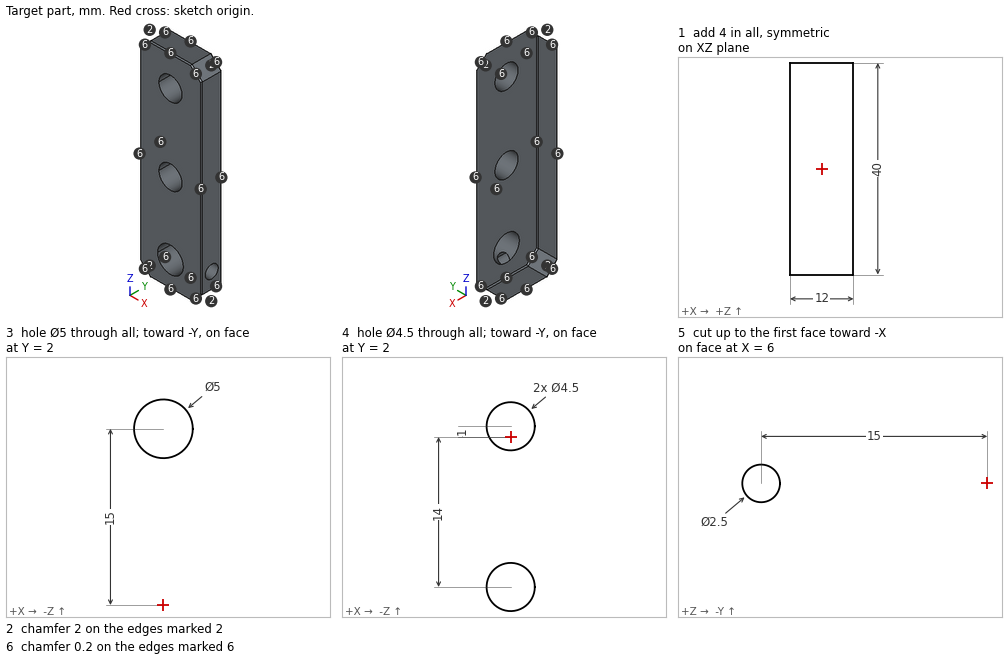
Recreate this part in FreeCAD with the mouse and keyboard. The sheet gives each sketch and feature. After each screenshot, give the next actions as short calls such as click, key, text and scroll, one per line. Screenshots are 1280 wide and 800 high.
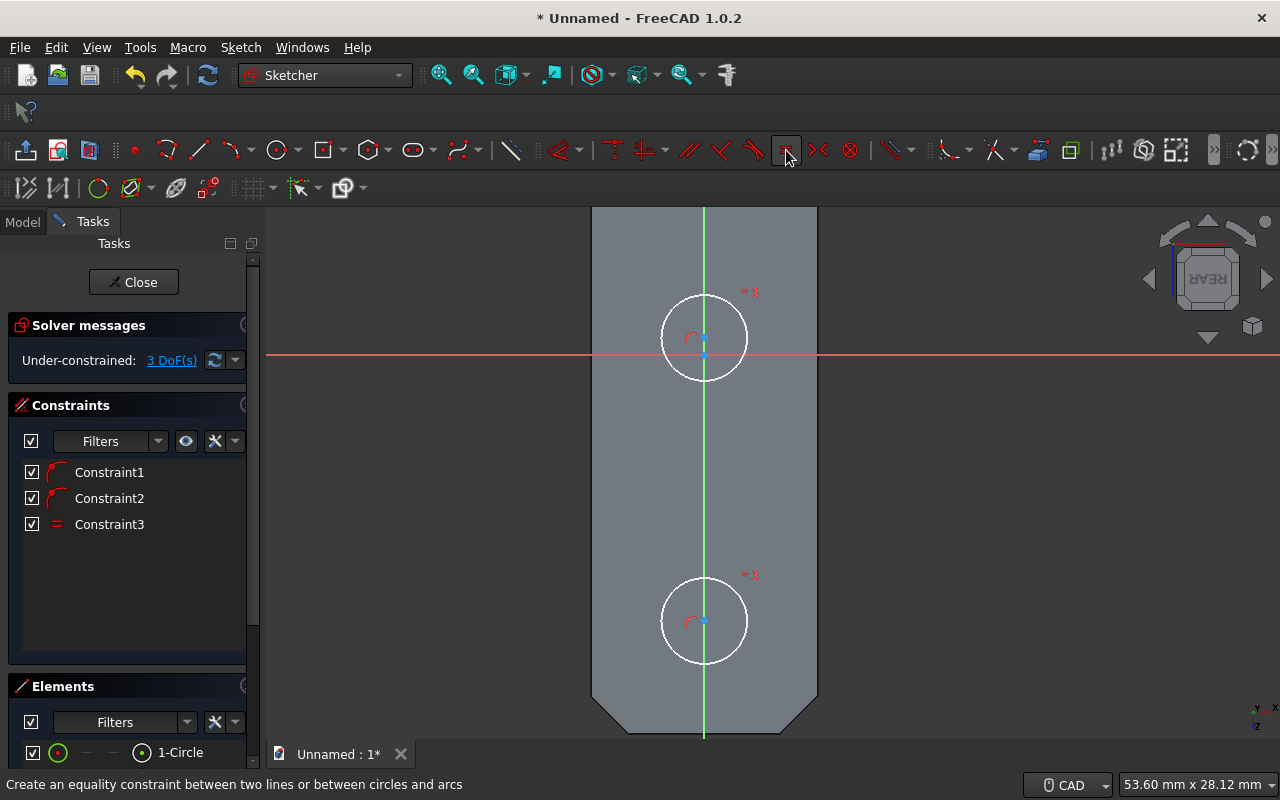
click(558, 150)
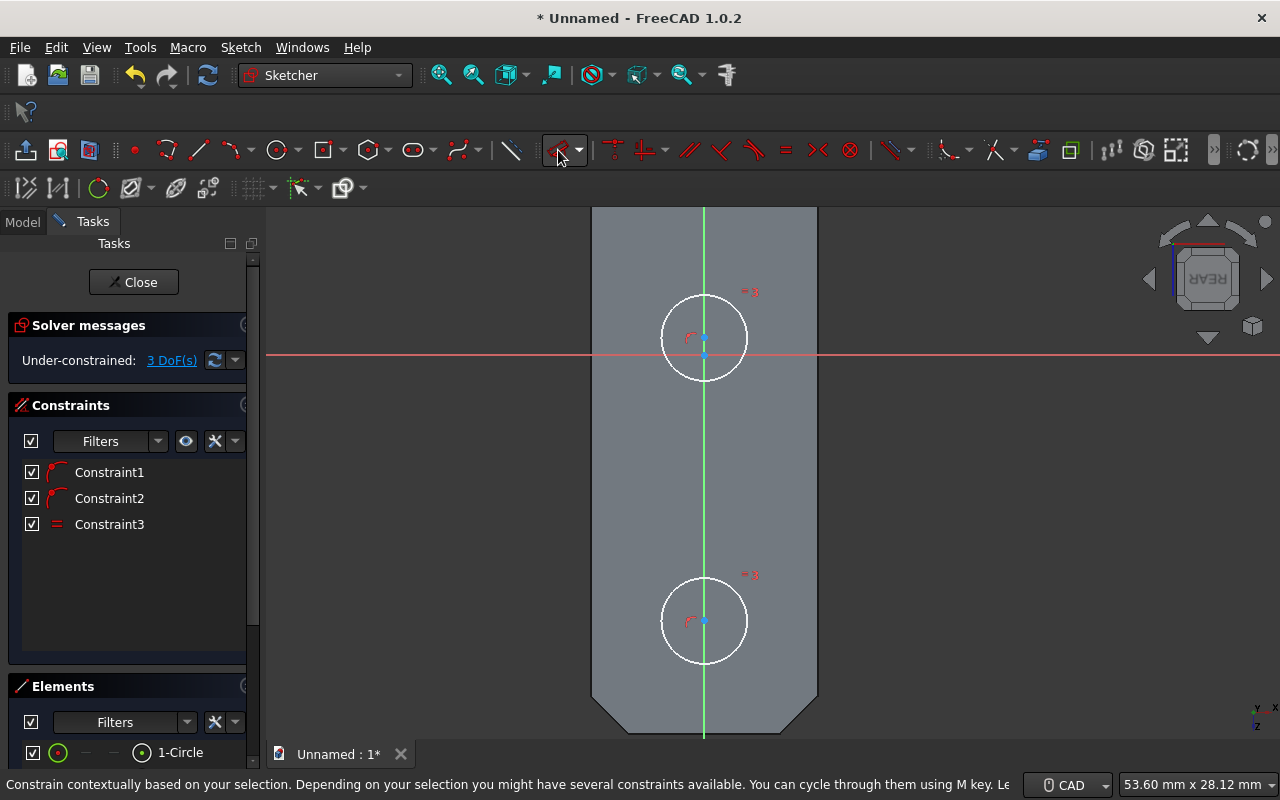
click(735, 308)
click(758, 286)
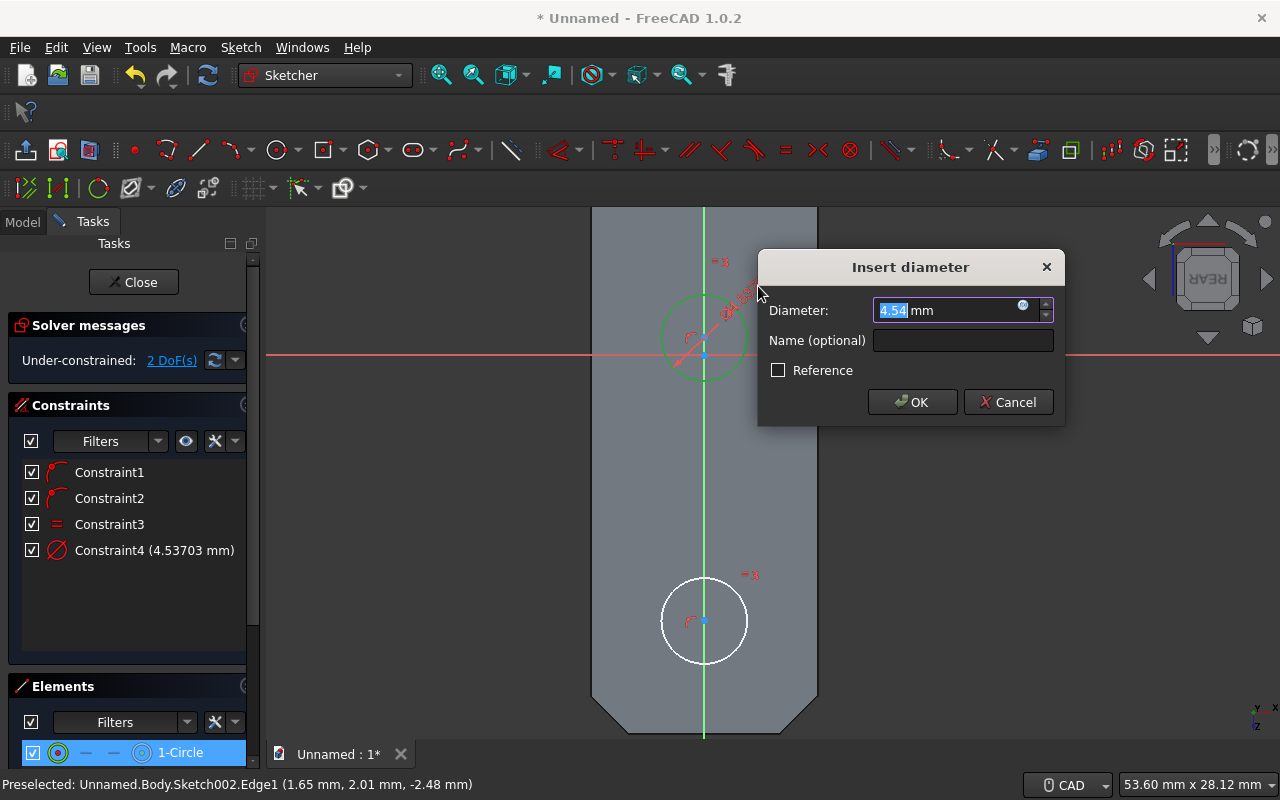
text(4.5)
key(Return)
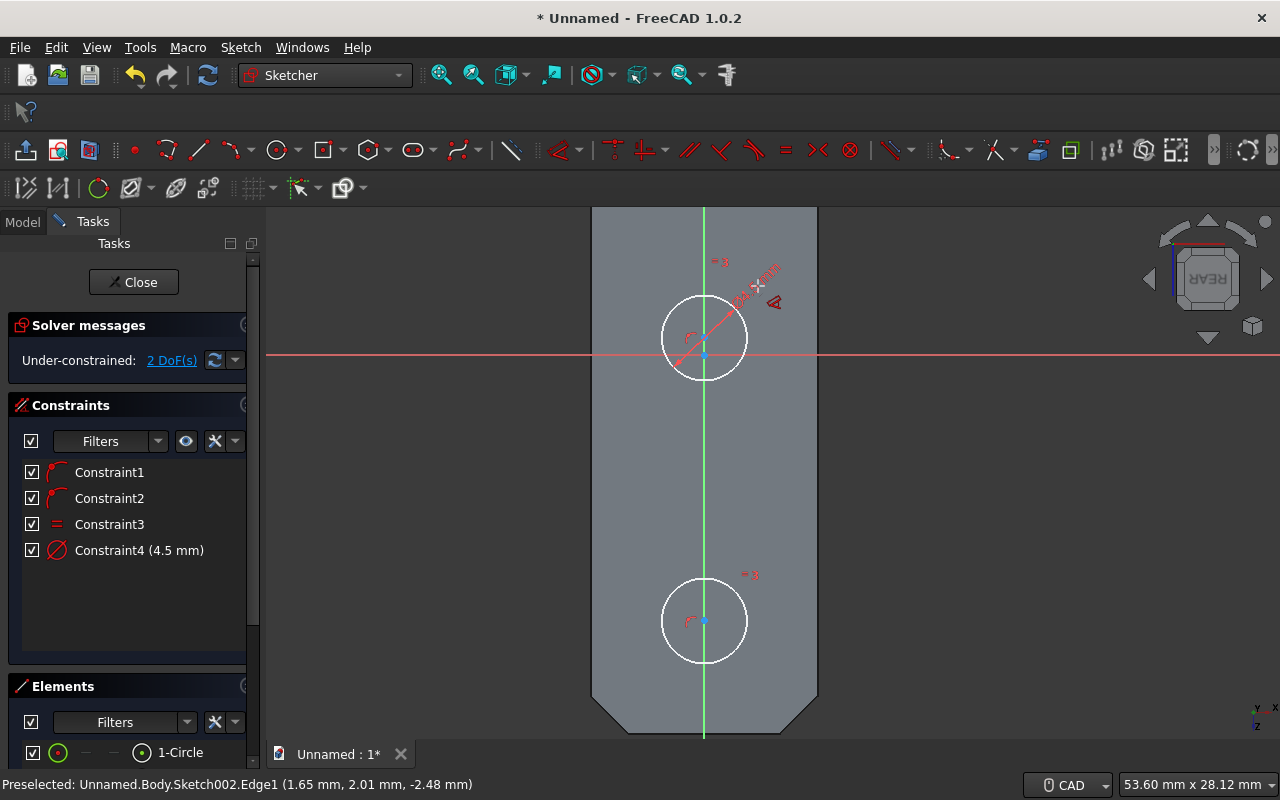
scroll(704, 338, up, 4)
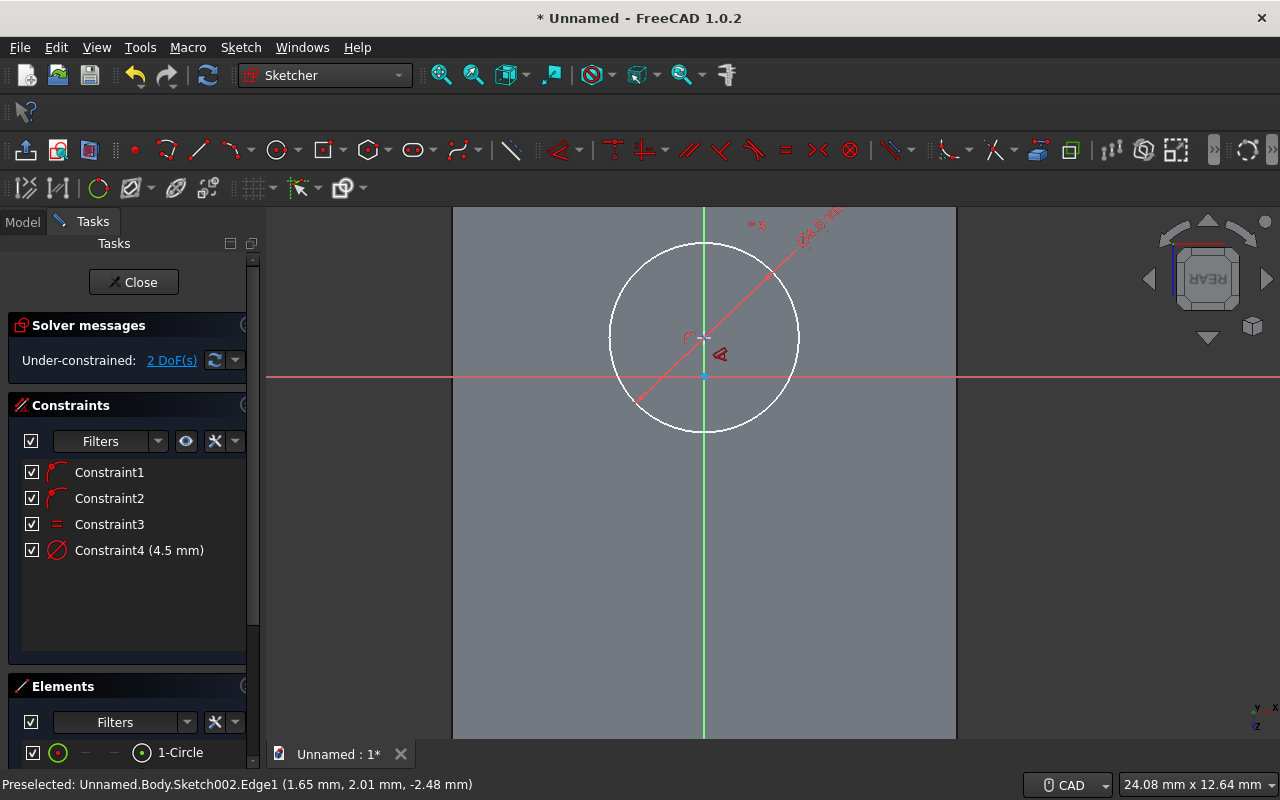
click(704, 338)
click(738, 357)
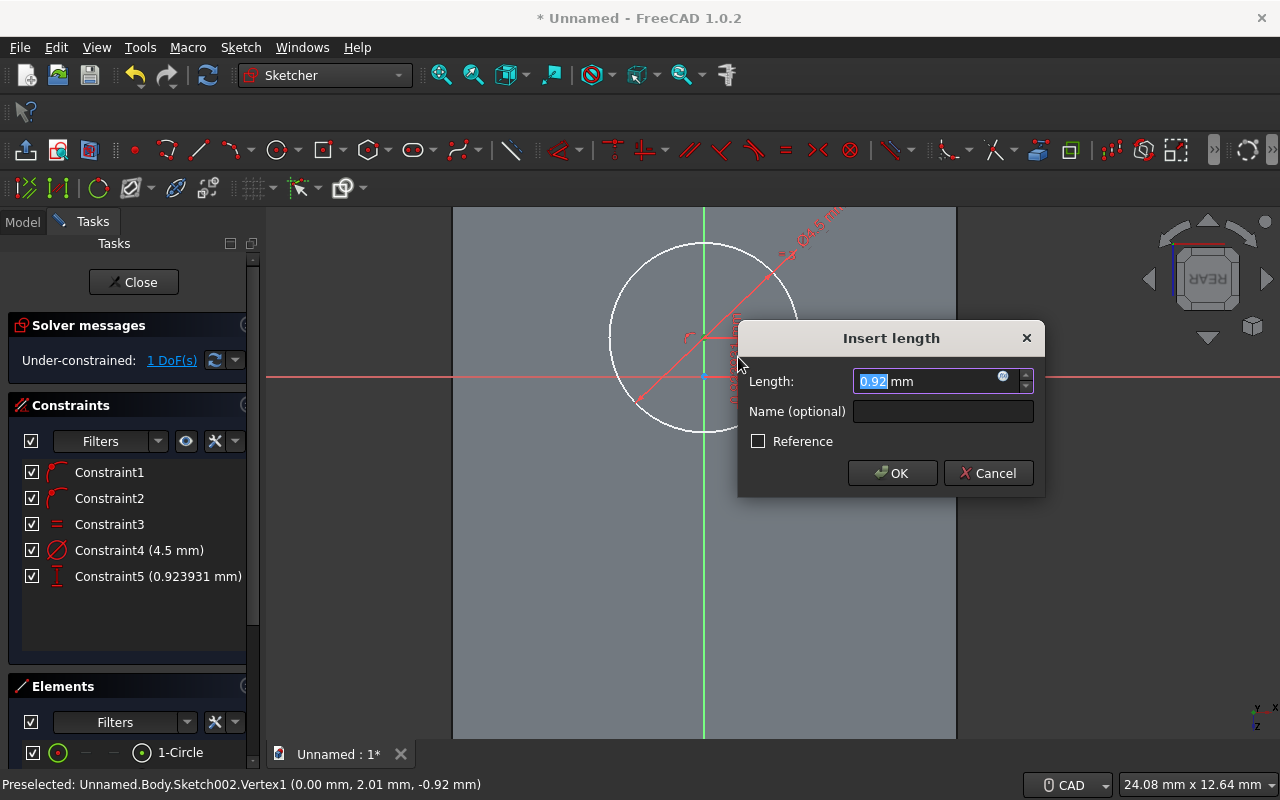
text(1)
key(Return)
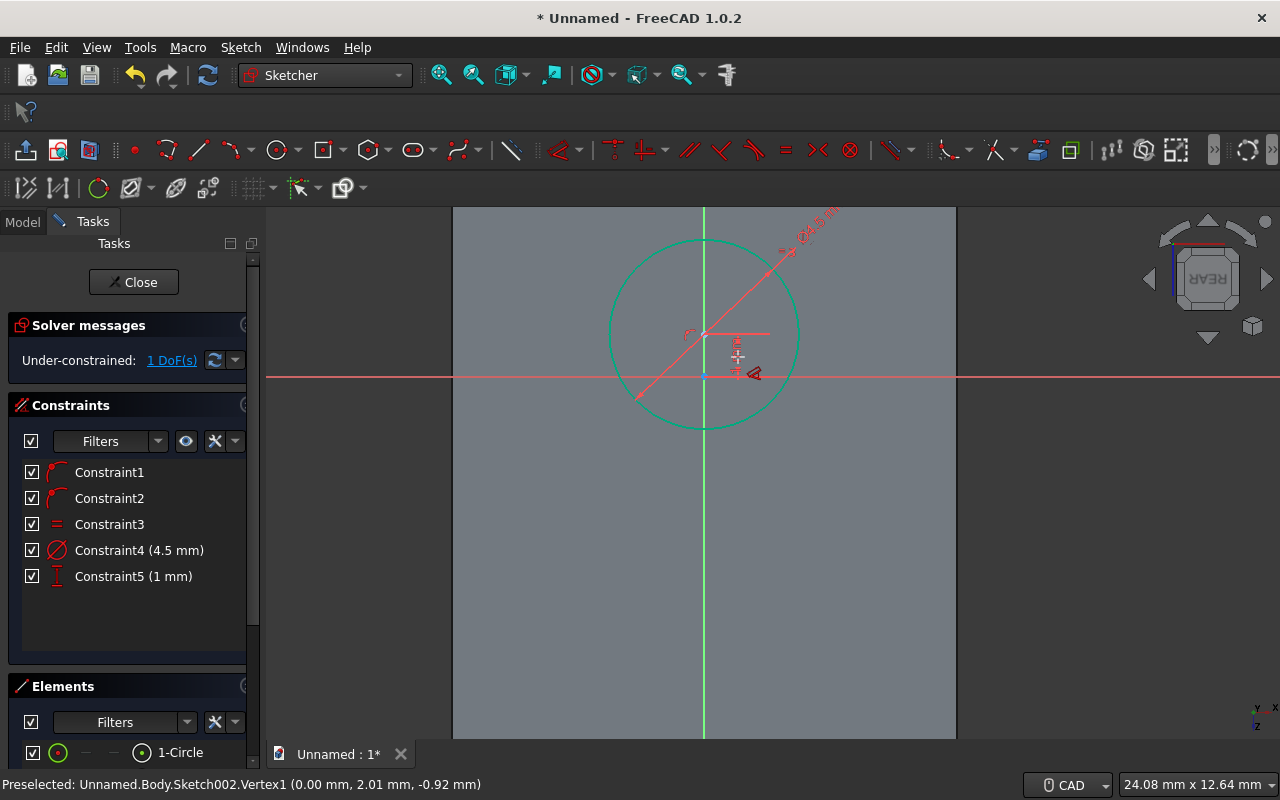
scroll(705, 328, down, 4)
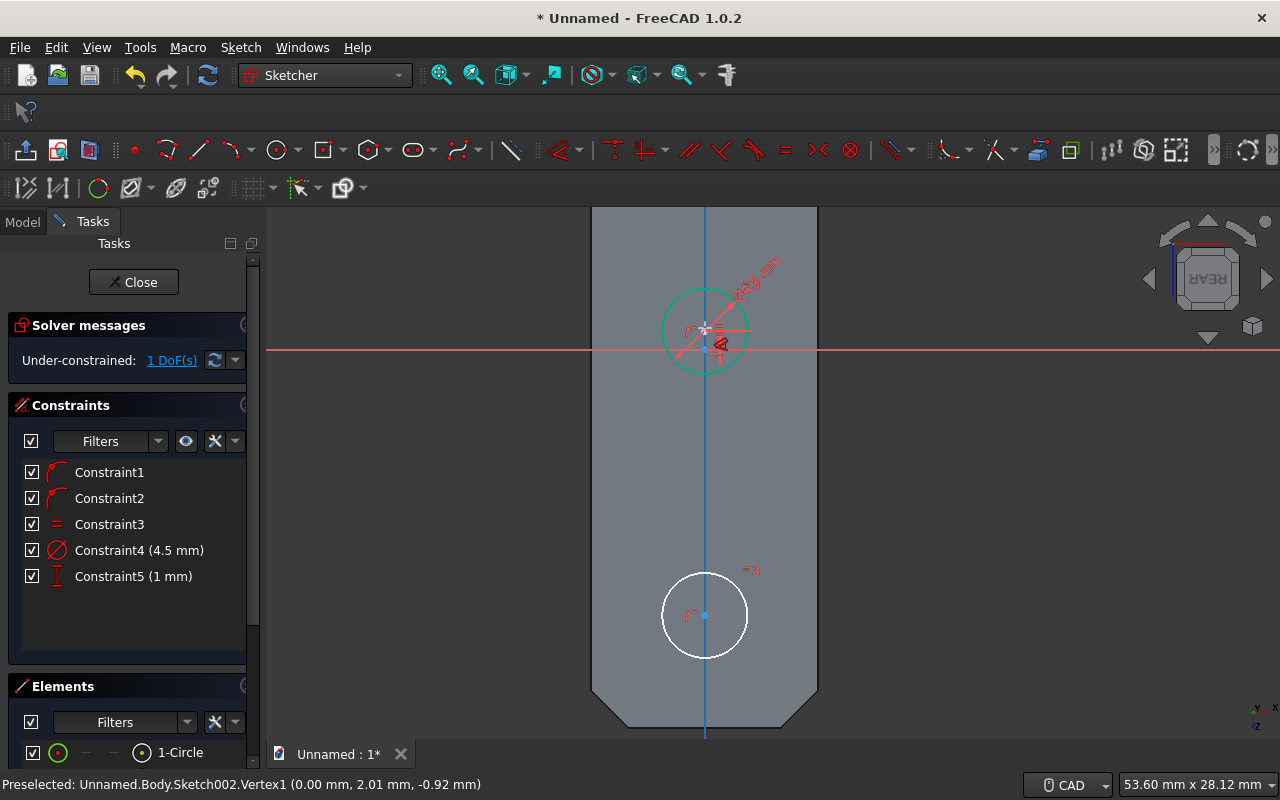
click(705, 615)
click(739, 483)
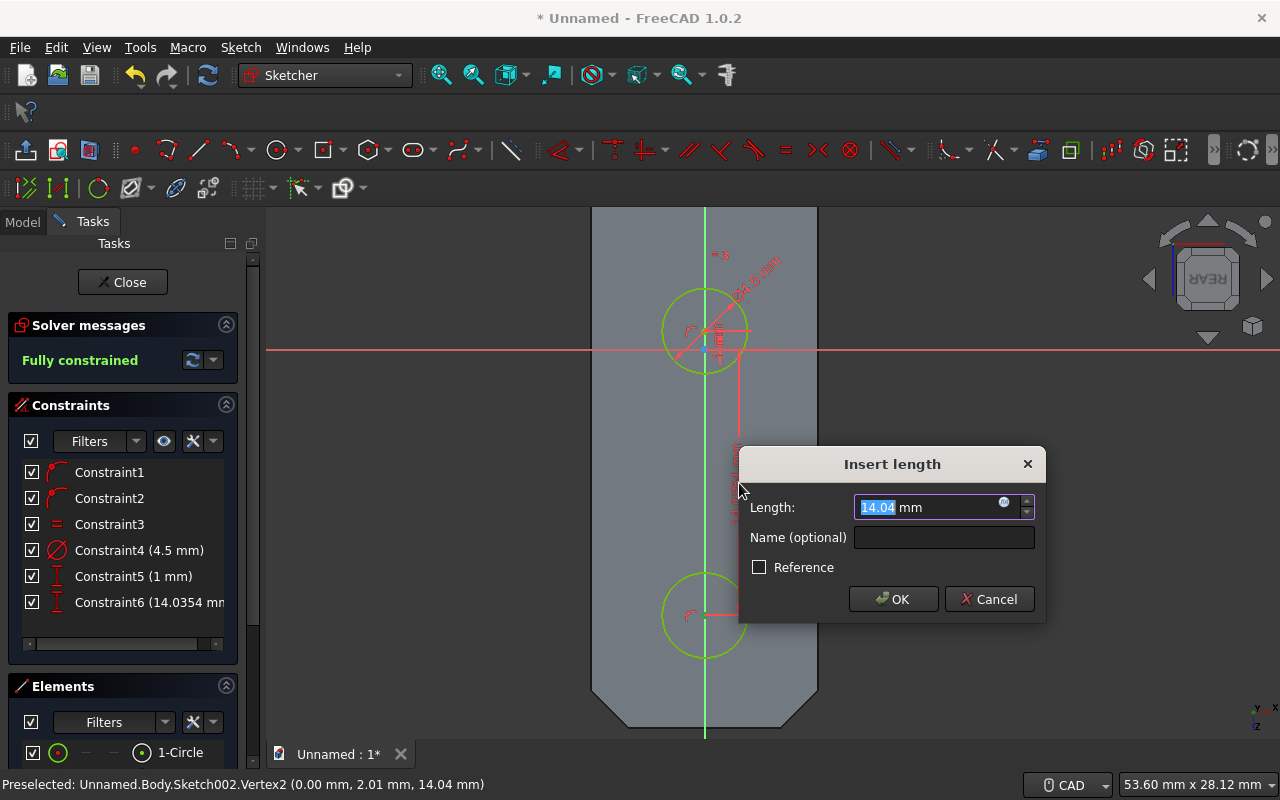
text(14)
key(Return)
key(Escape)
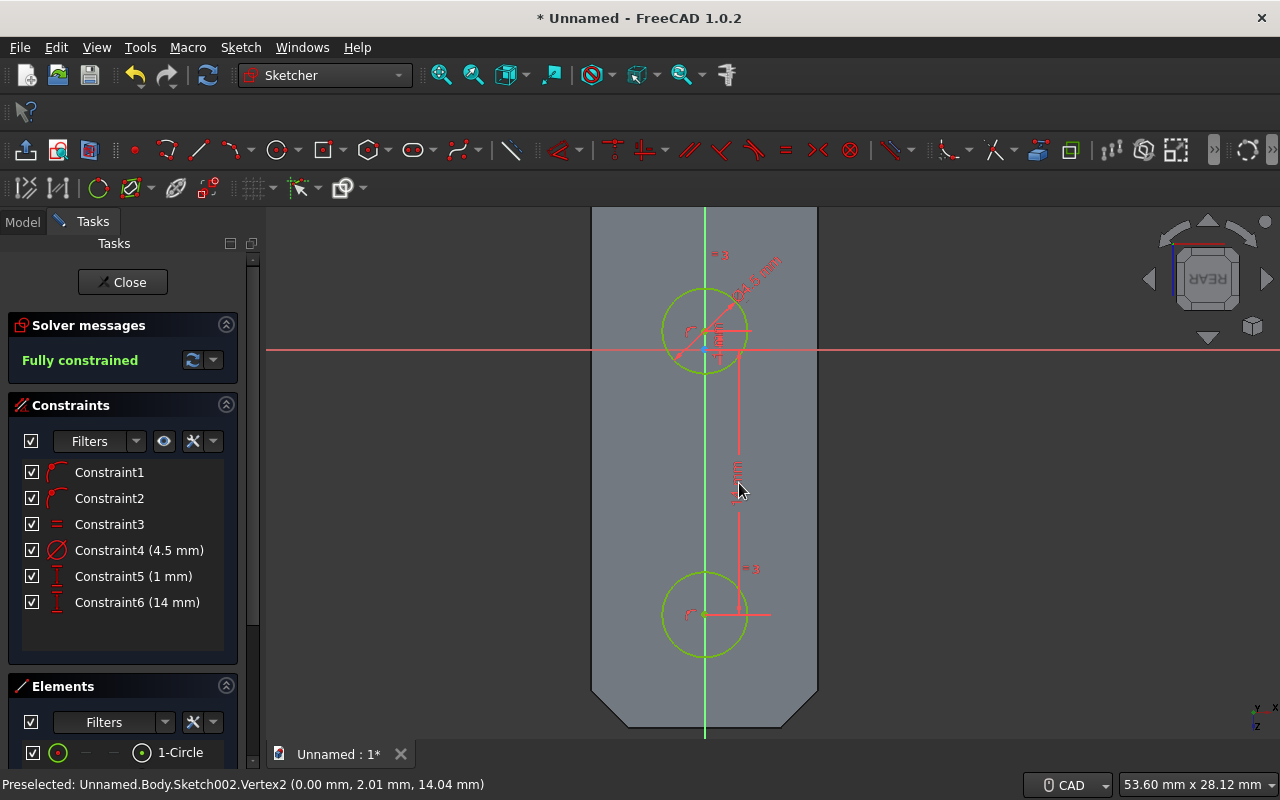
click(123, 282)